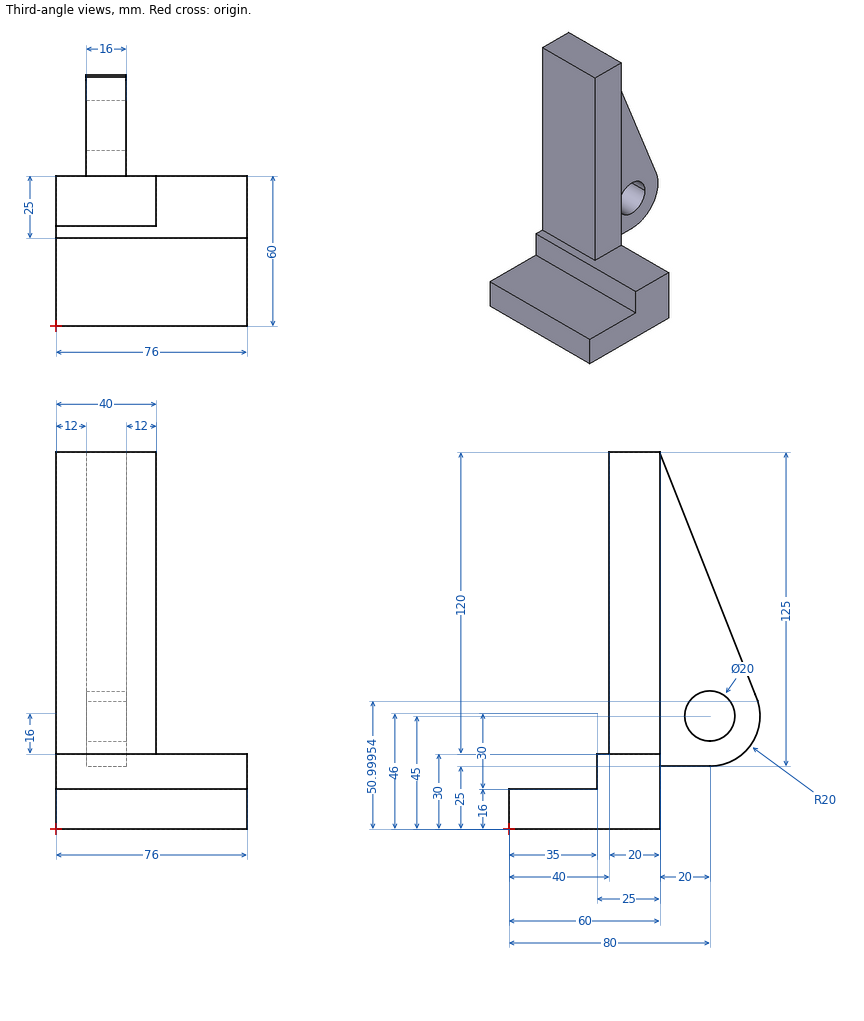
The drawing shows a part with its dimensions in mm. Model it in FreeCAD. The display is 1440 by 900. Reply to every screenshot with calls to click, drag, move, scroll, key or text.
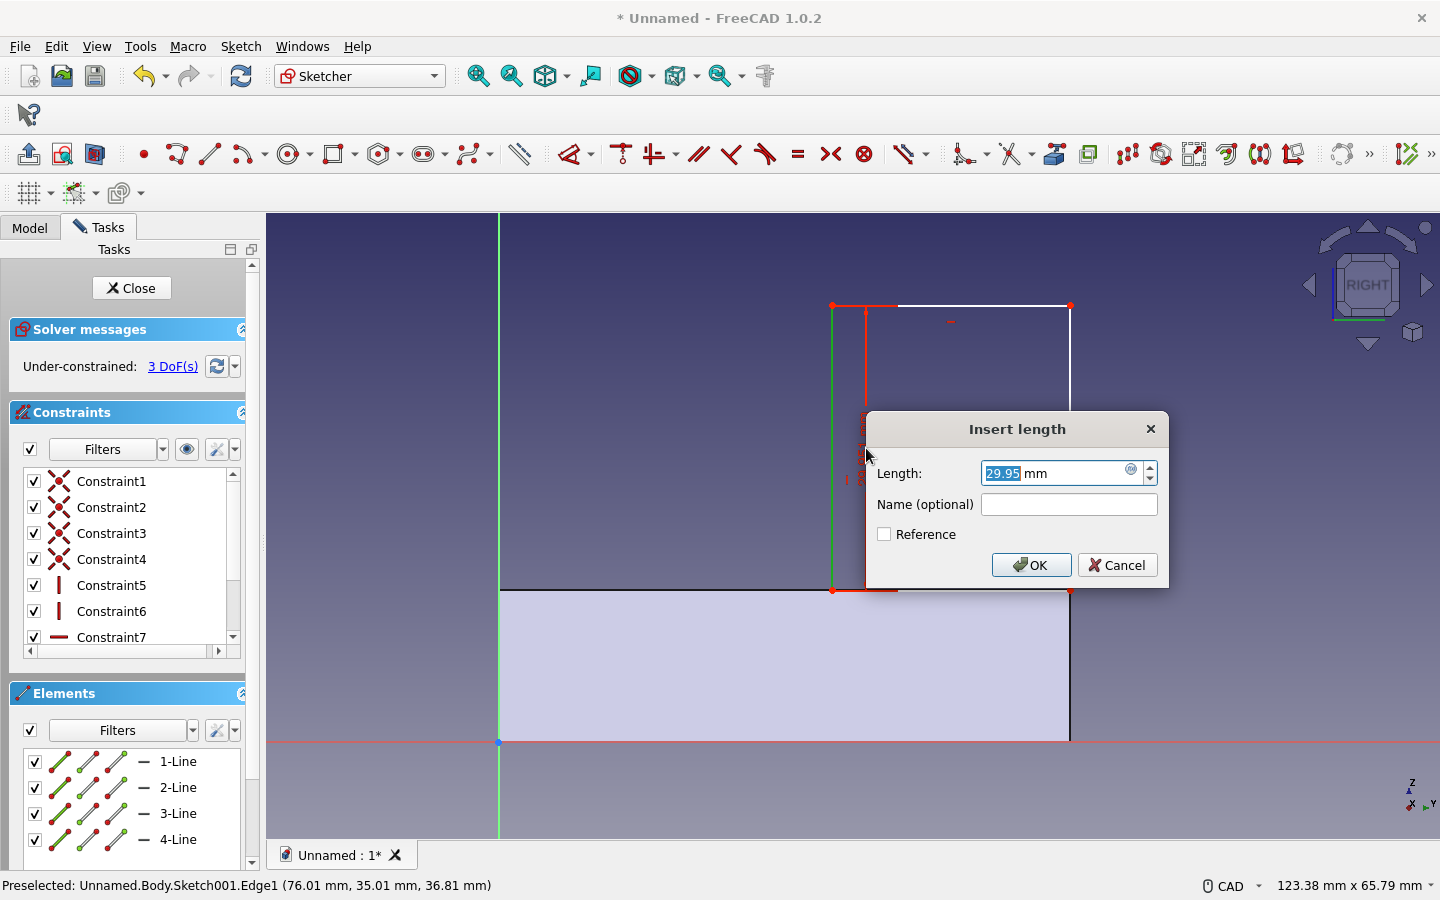
text(30)
key(Return)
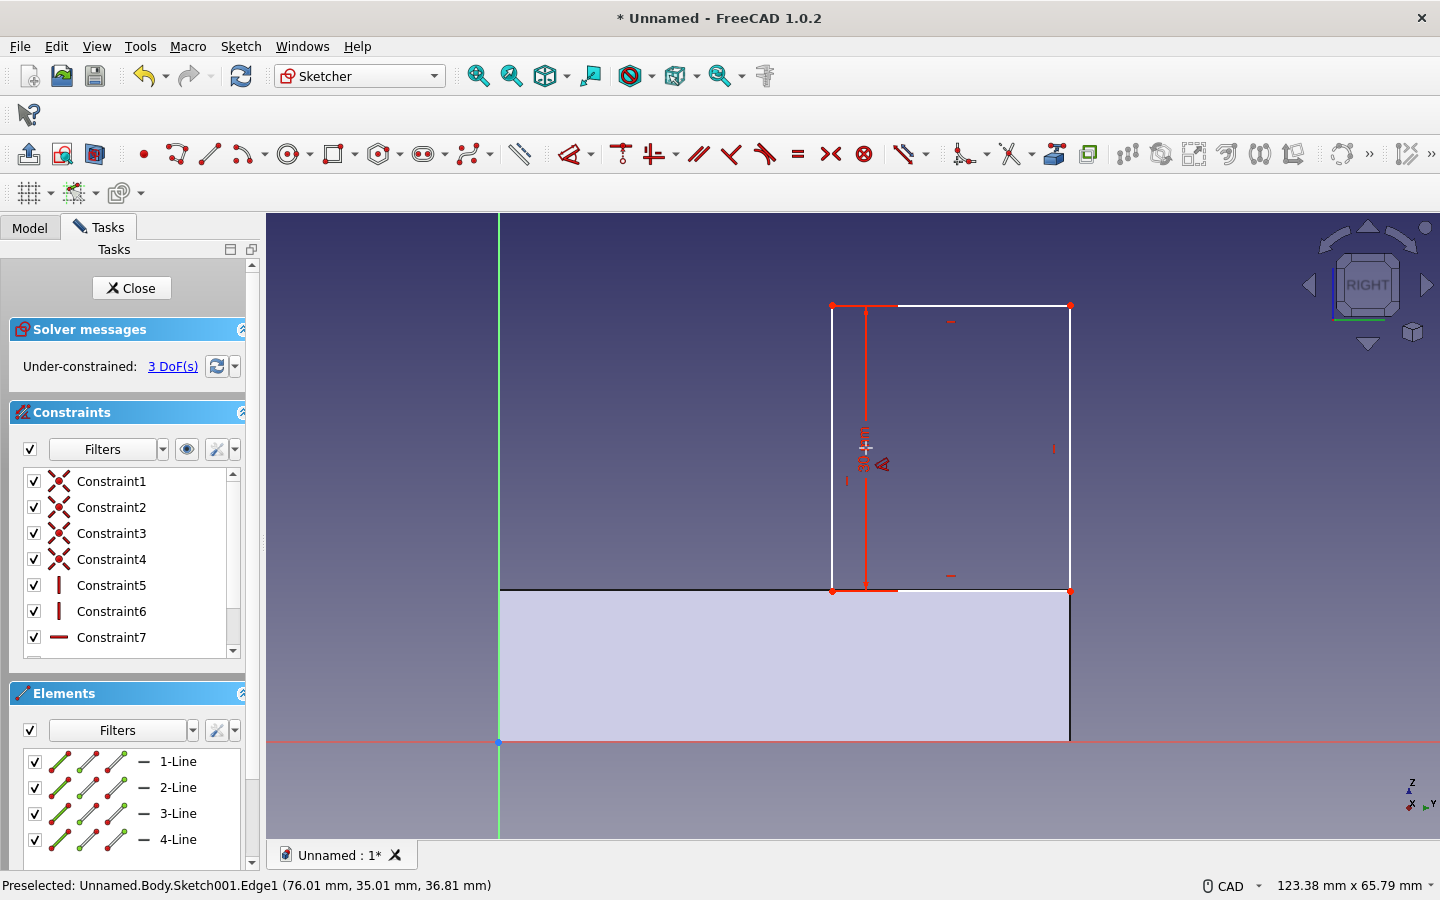
click(903, 591)
click(951, 625)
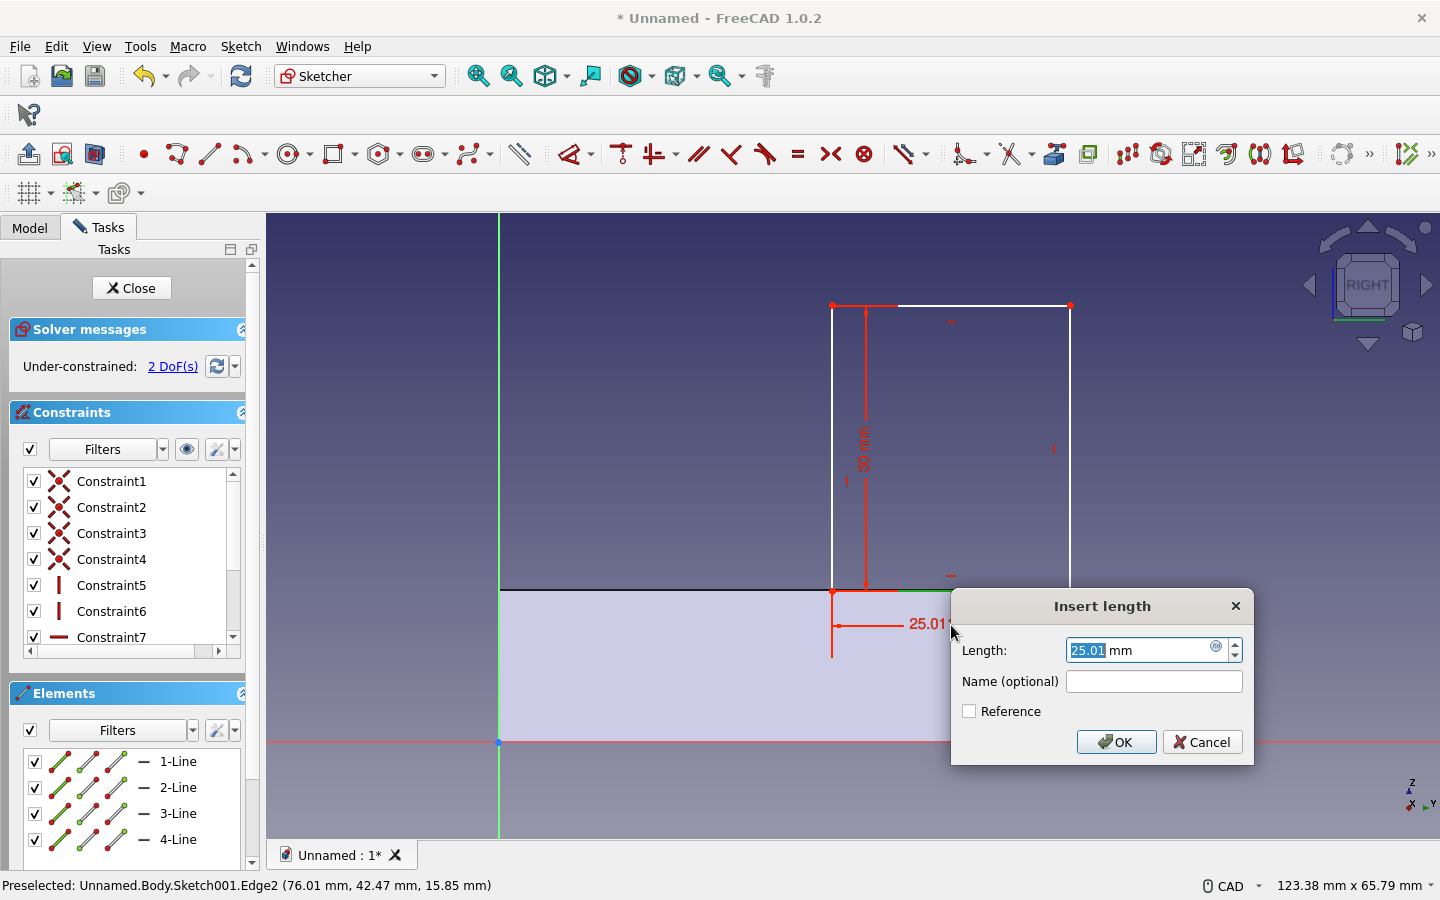
text(25)
key(Return)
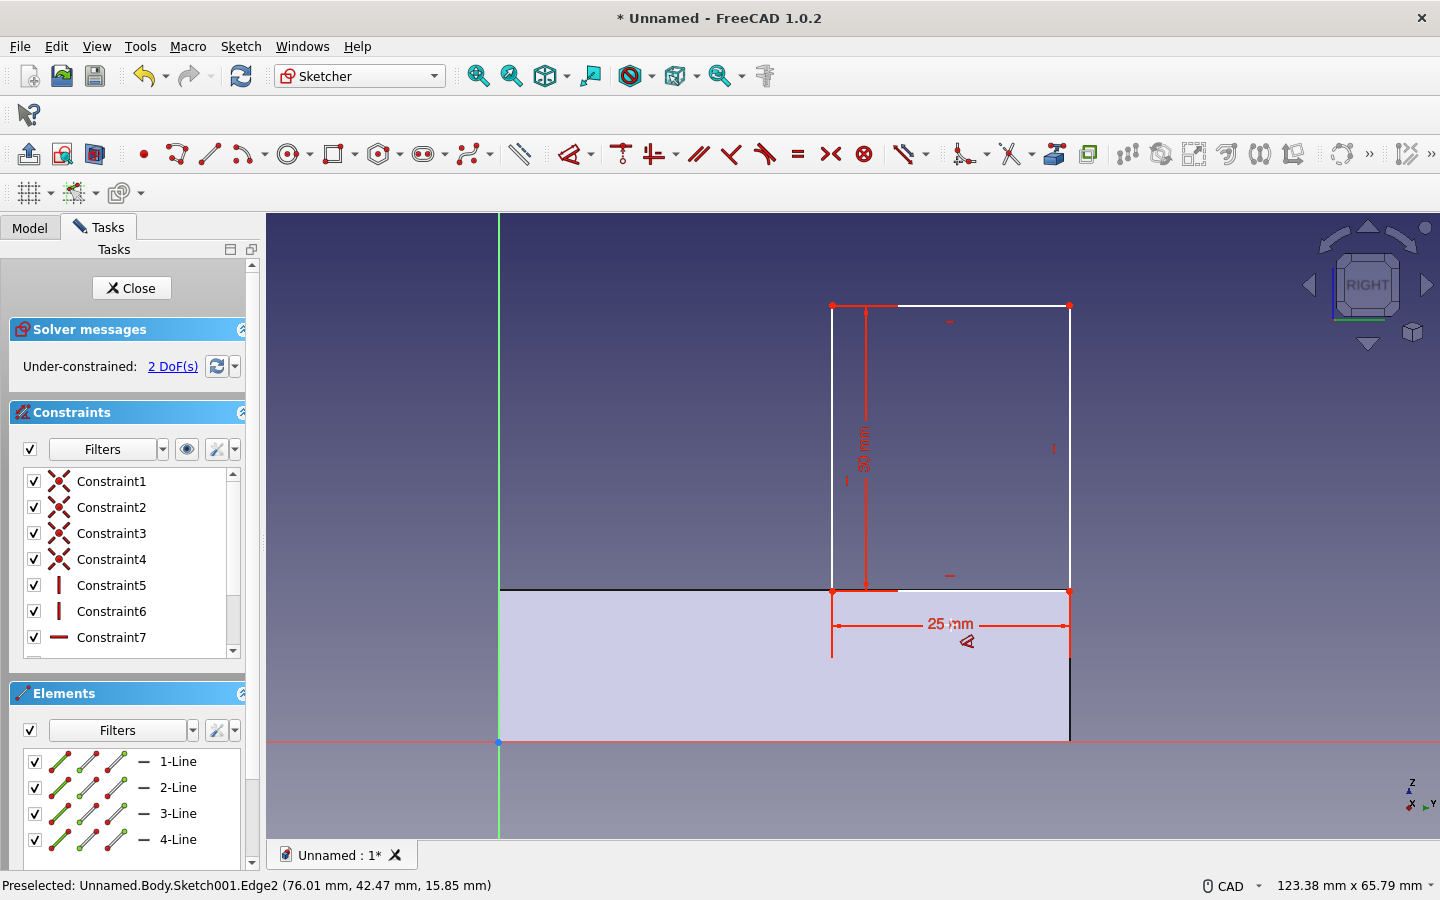
click(832, 306)
click(665, 776)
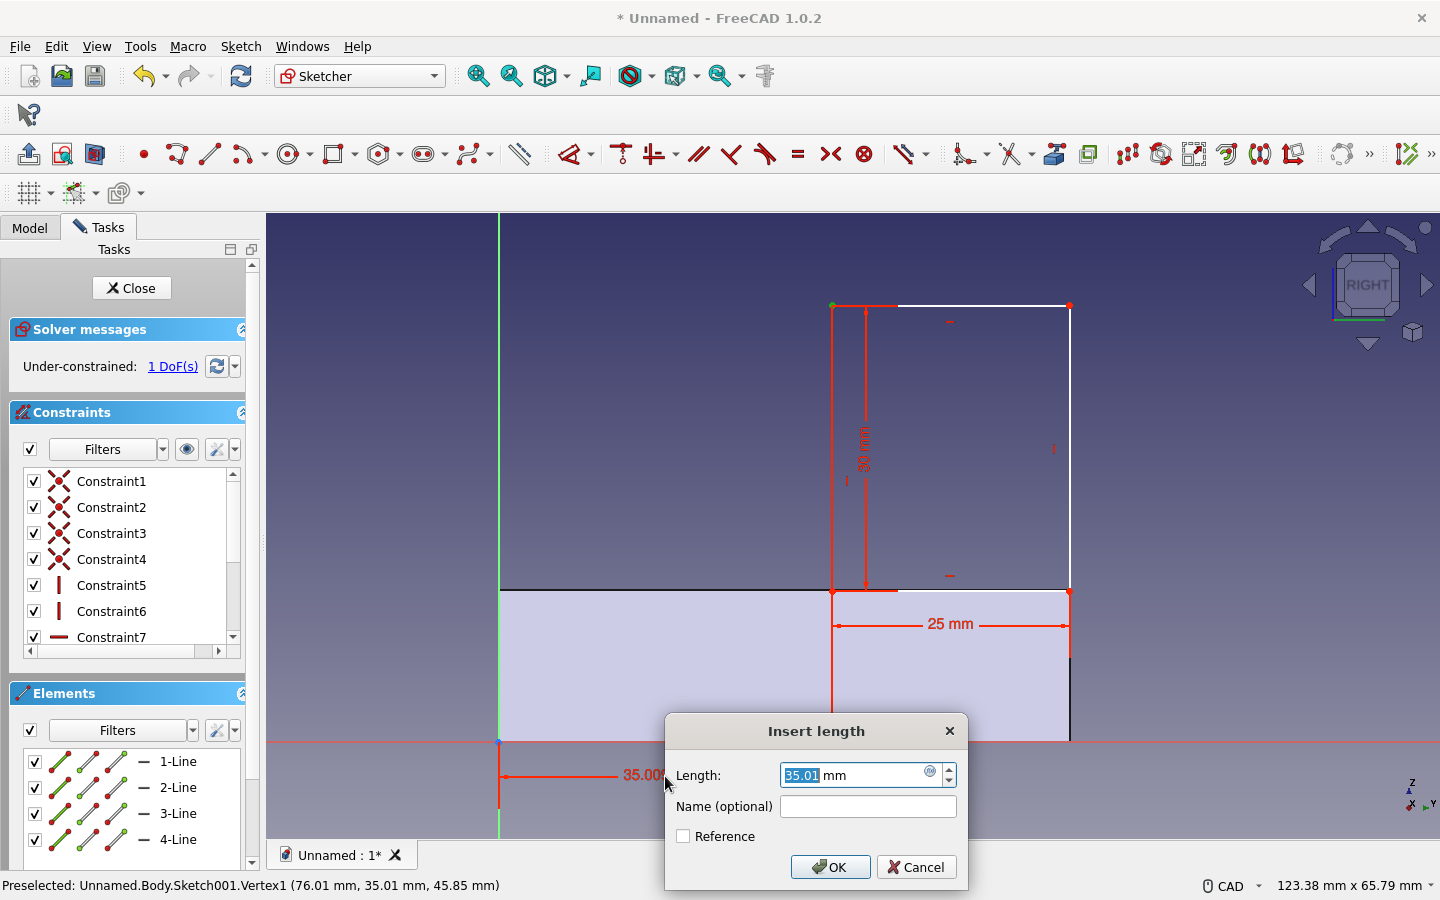
text(35)
key(Return)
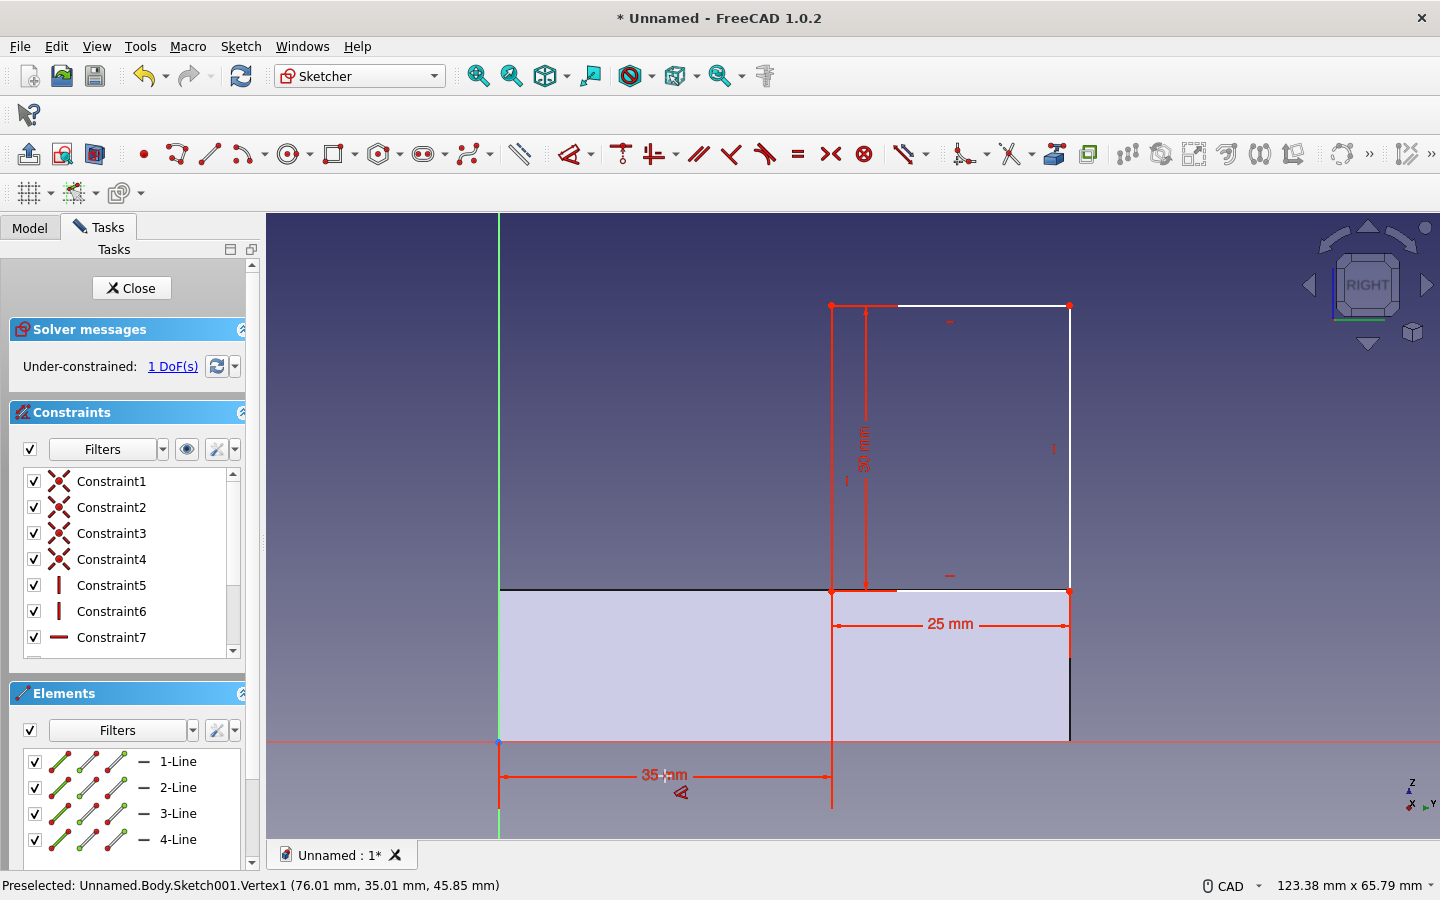
click(832, 306)
click(465, 524)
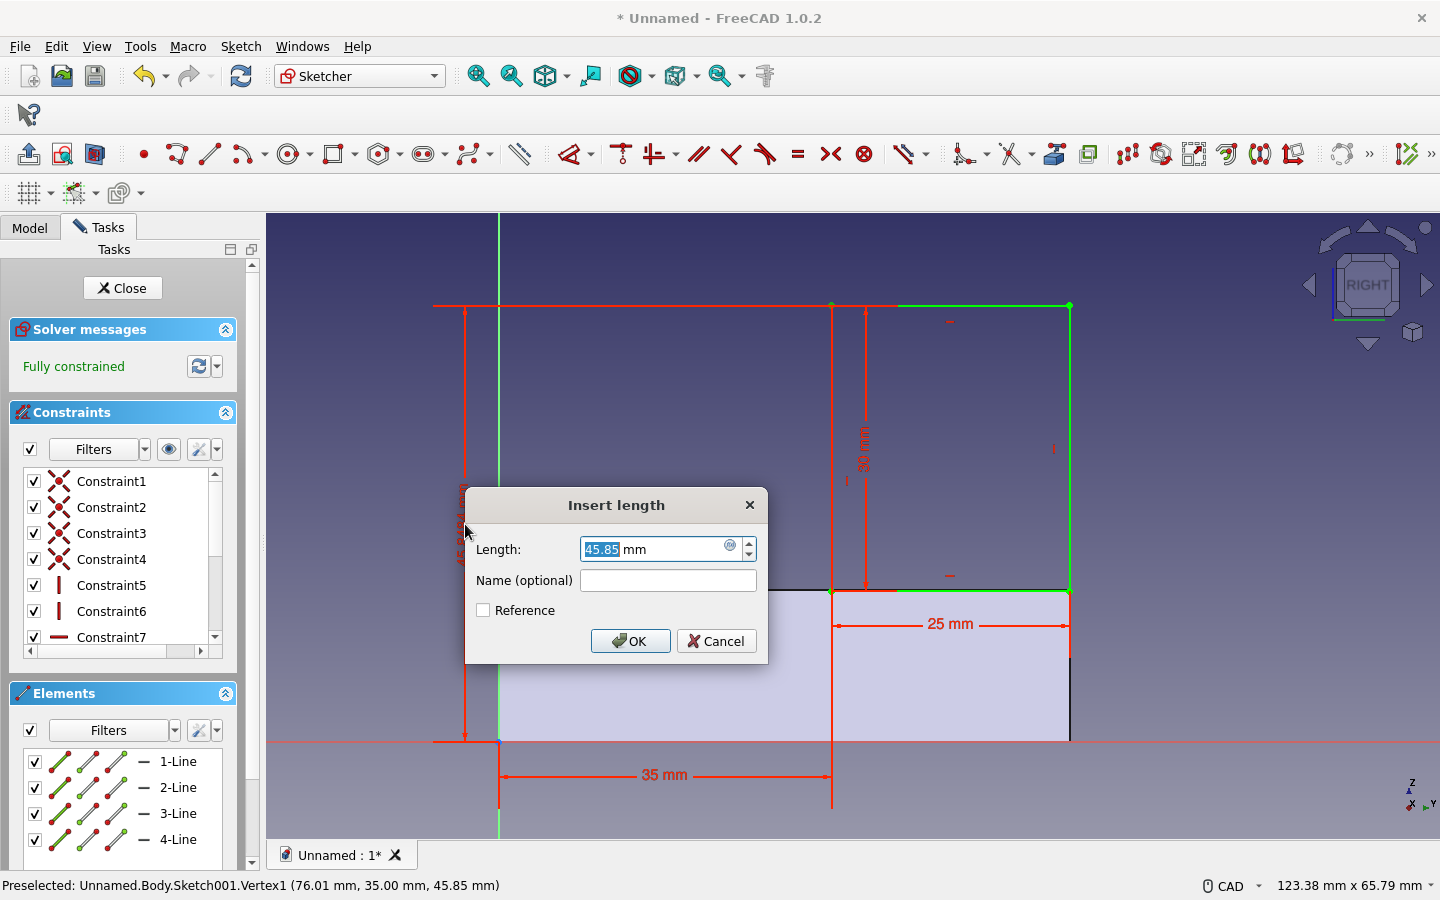
text(46)
key(Return)
key(Escape)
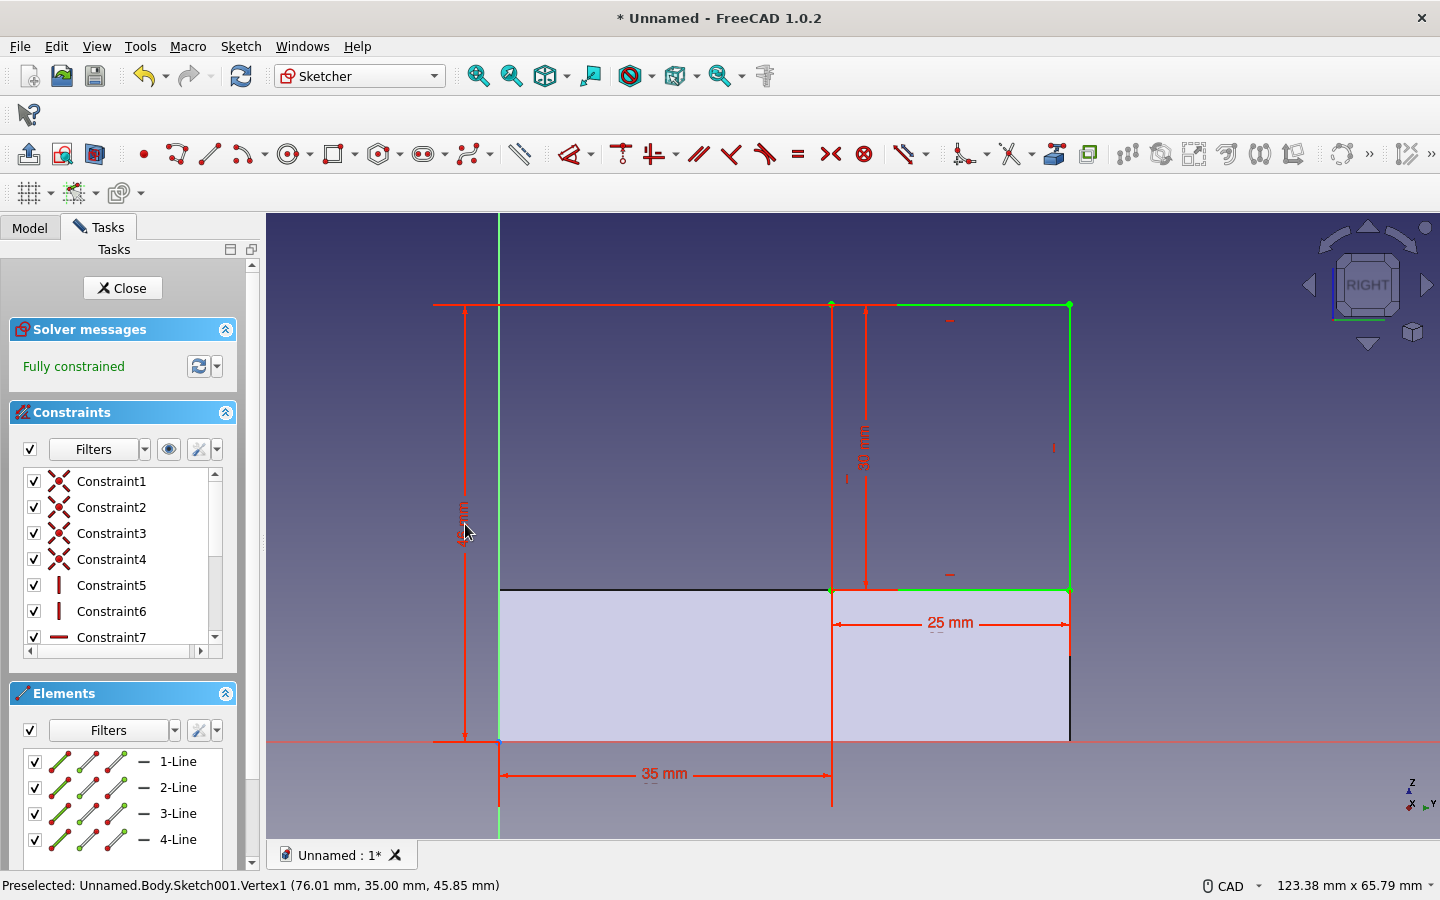
click(123, 288)